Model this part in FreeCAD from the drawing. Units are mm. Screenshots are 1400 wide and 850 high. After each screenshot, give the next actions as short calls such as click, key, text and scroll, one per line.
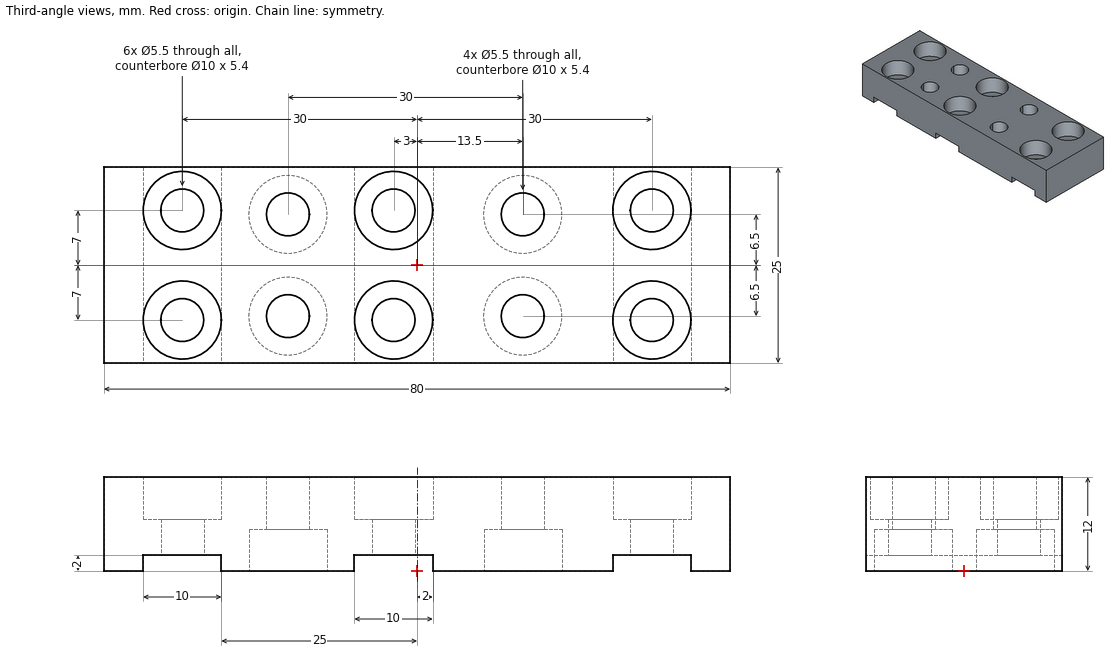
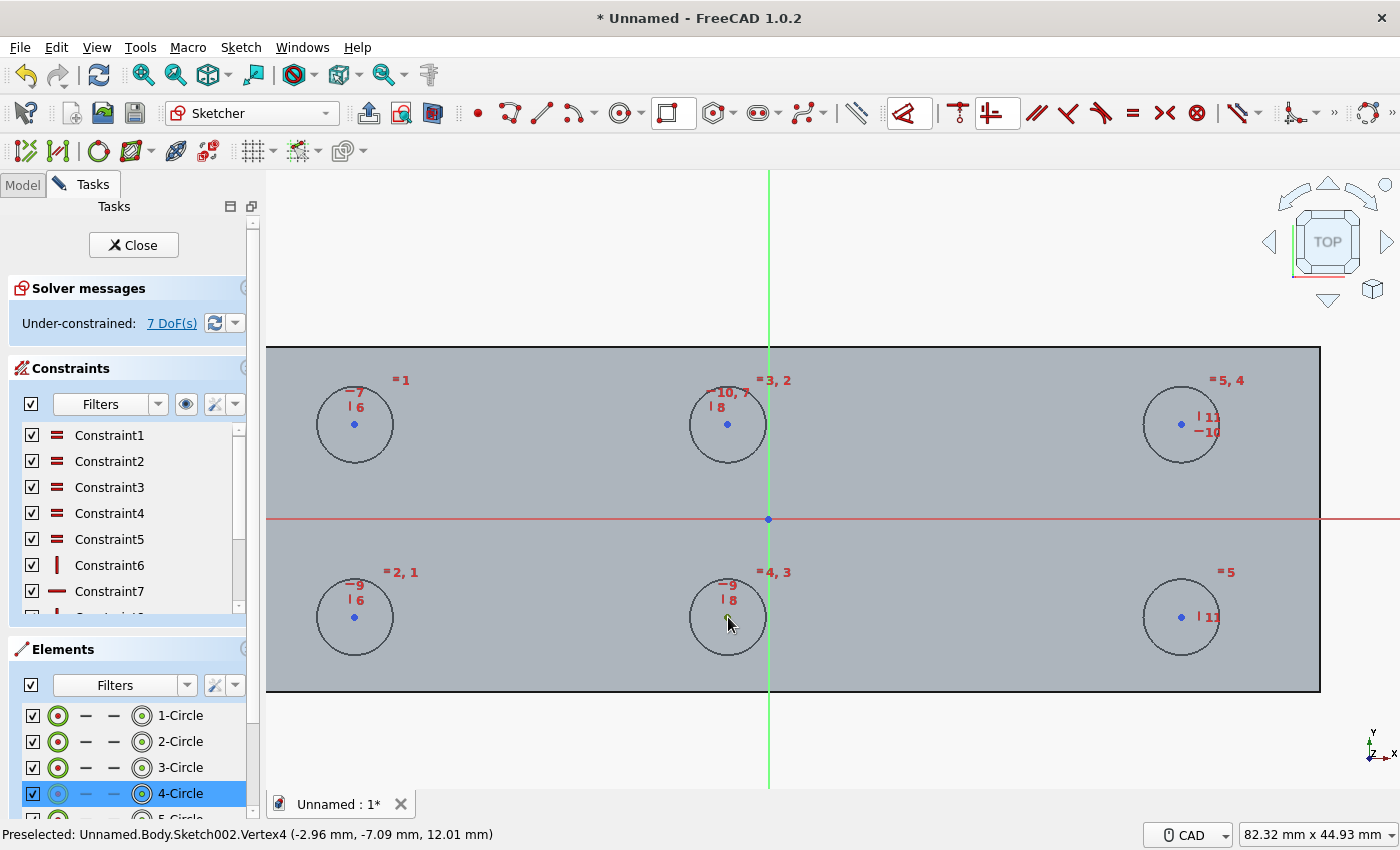
click(1181, 617)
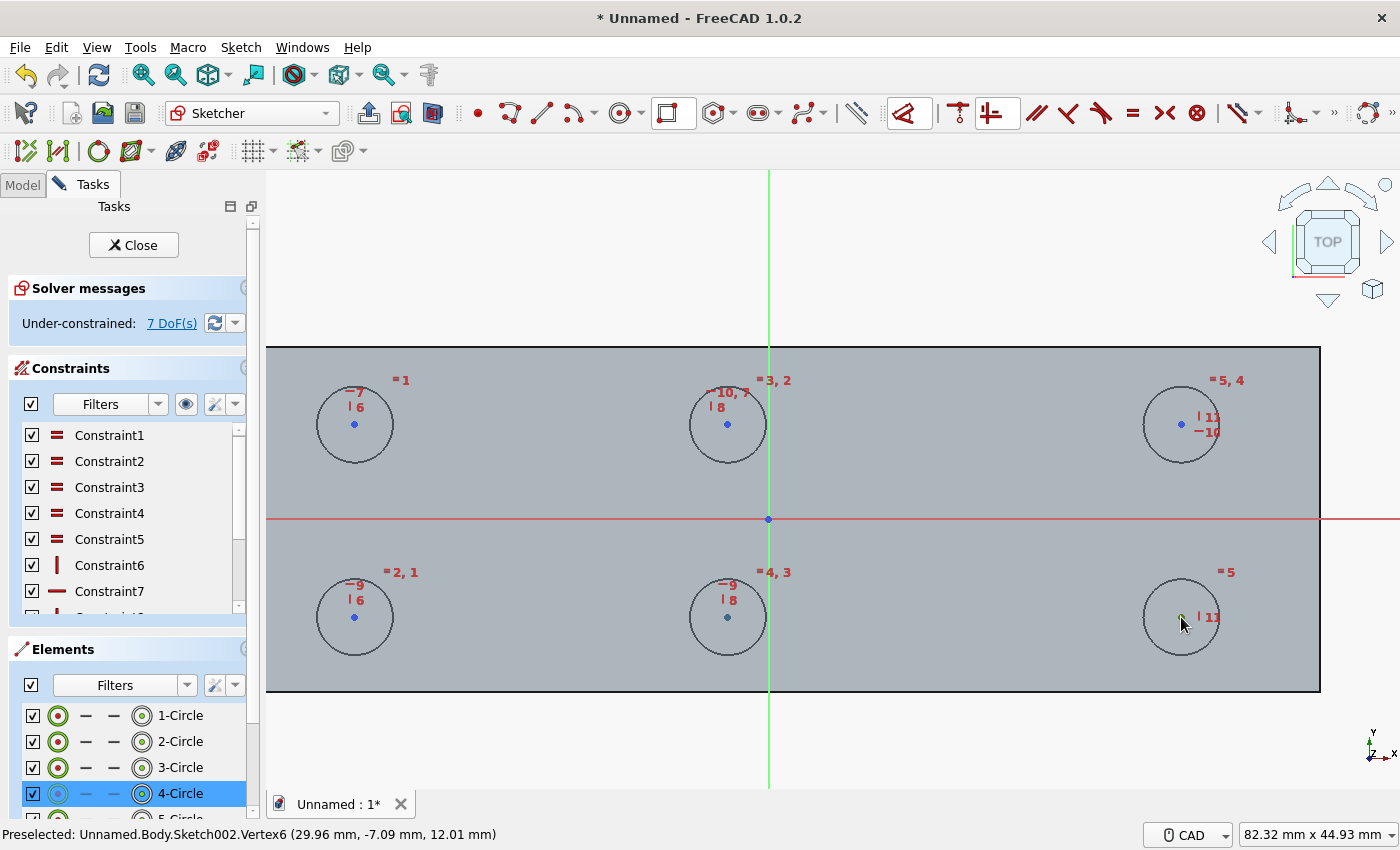
click(1014, 114)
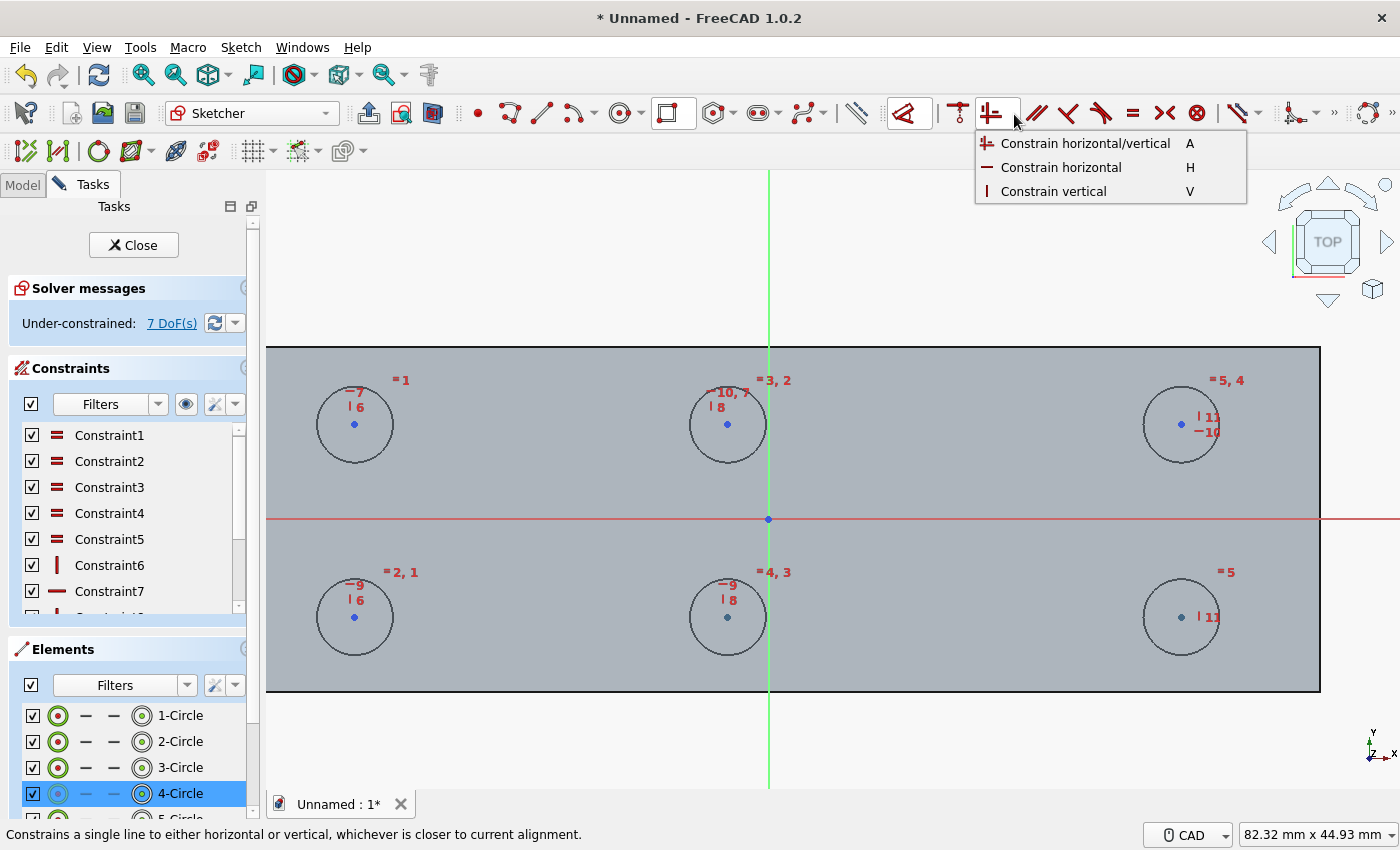
click(1111, 167)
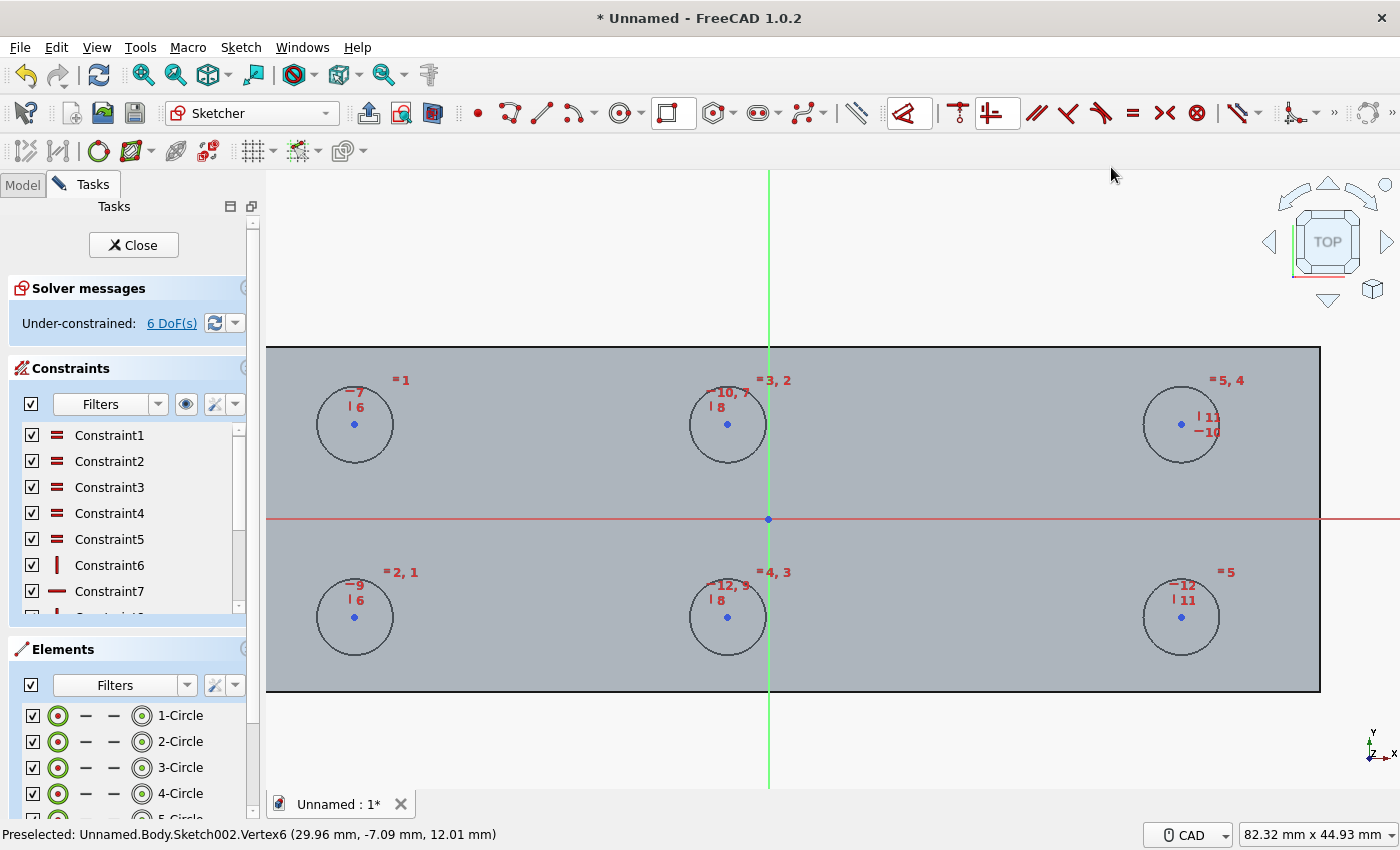
click(382, 398)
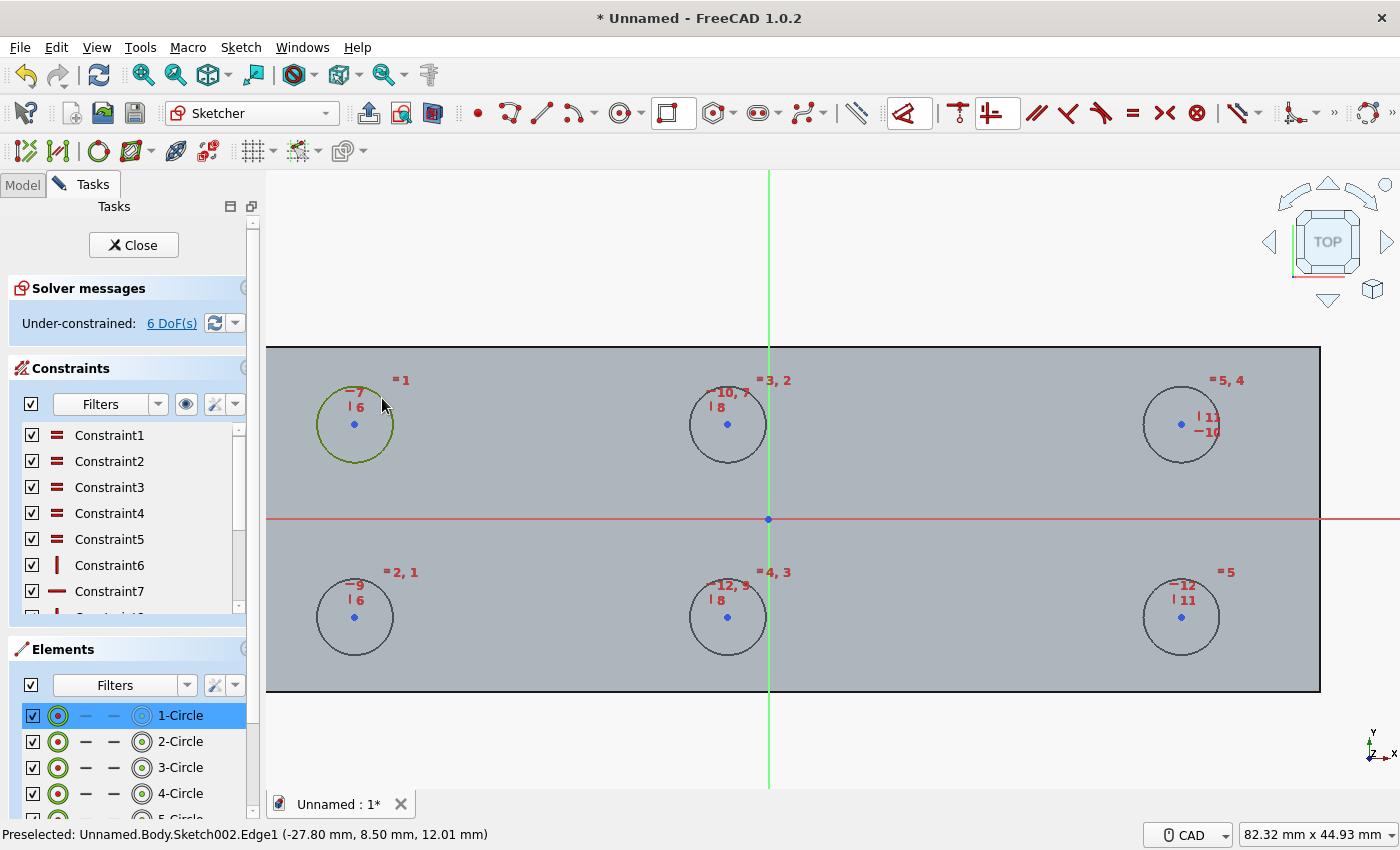
click(926, 114)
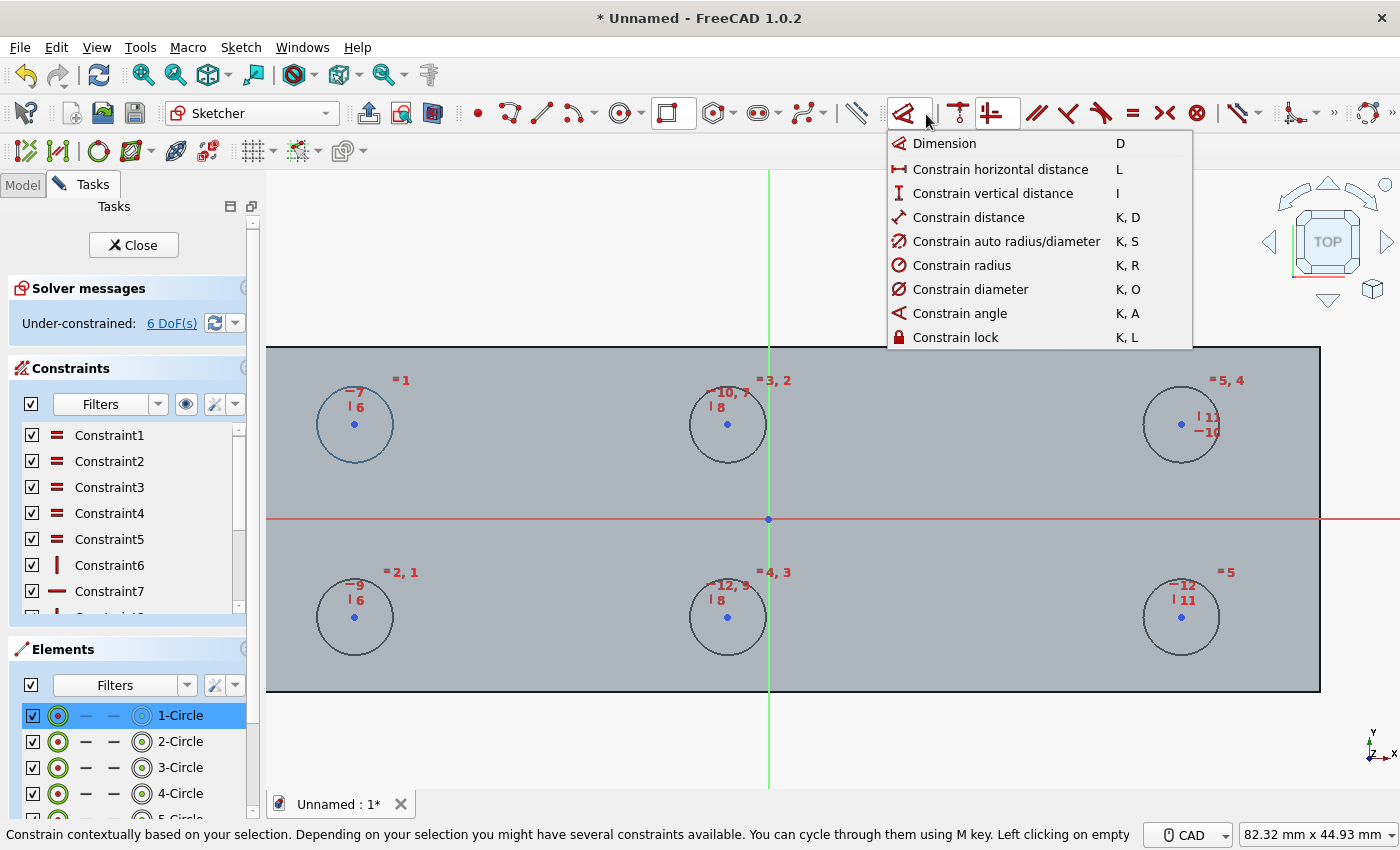
click(1040, 289)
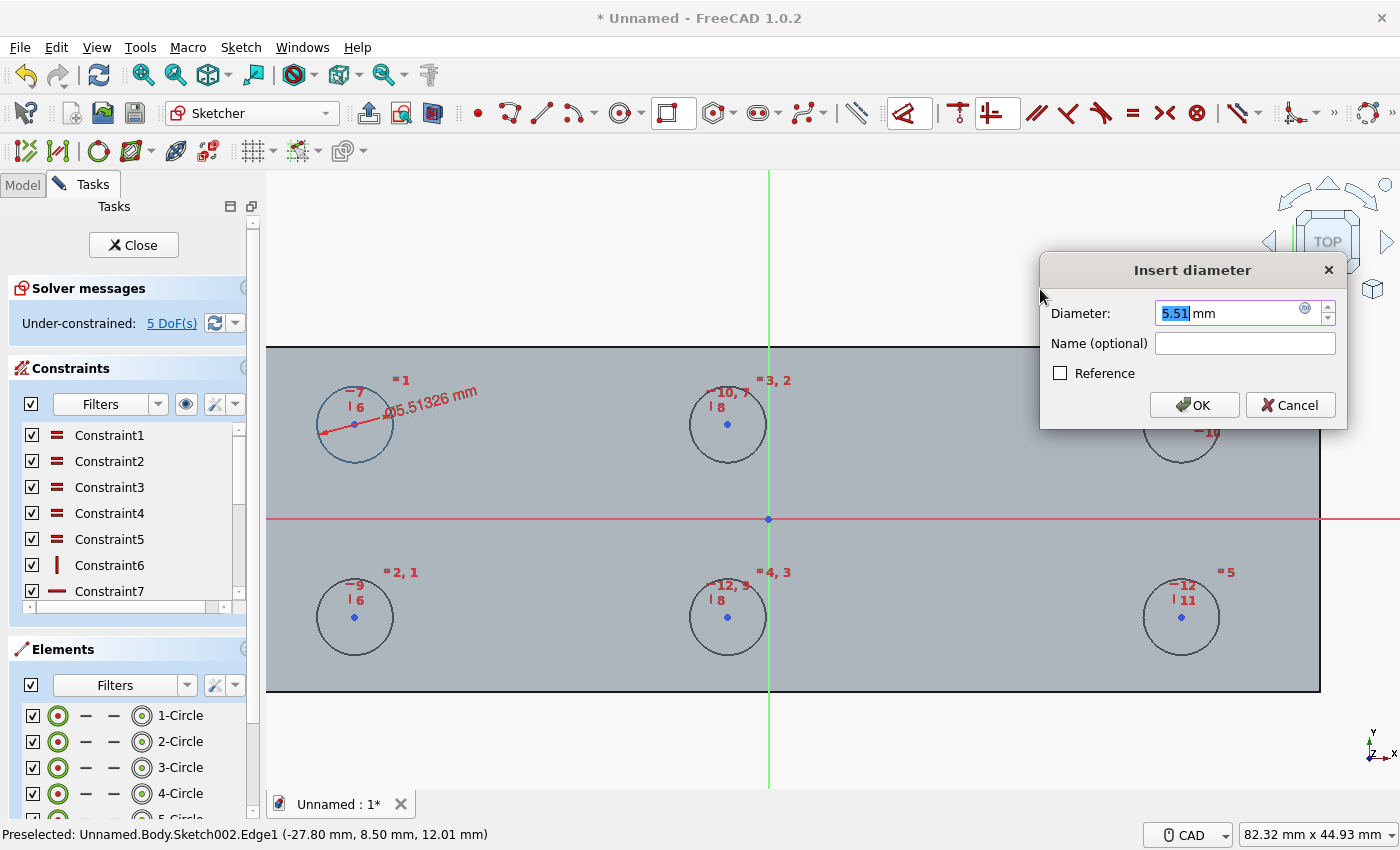
text(5.5)
key(Return)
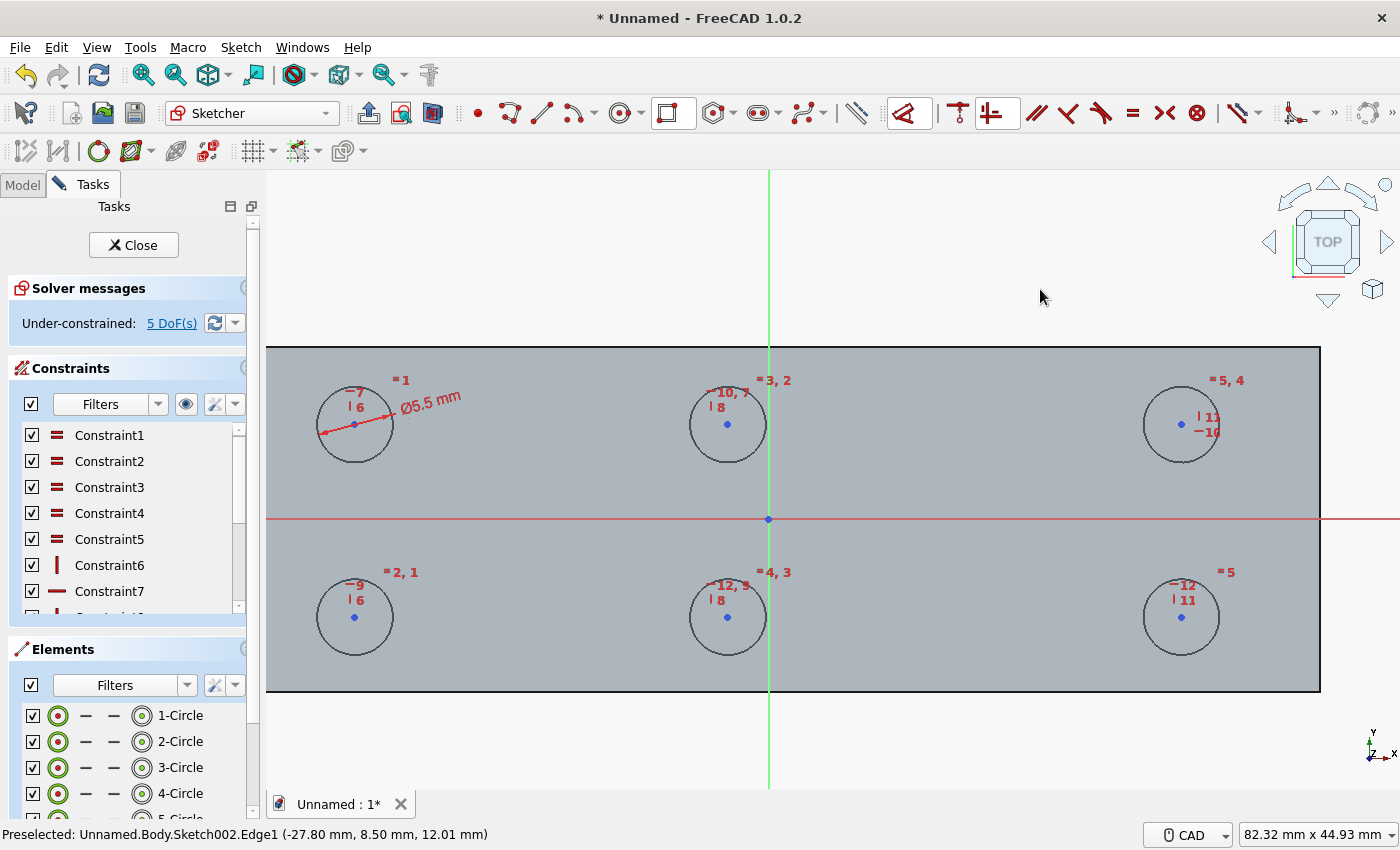
click(355, 425)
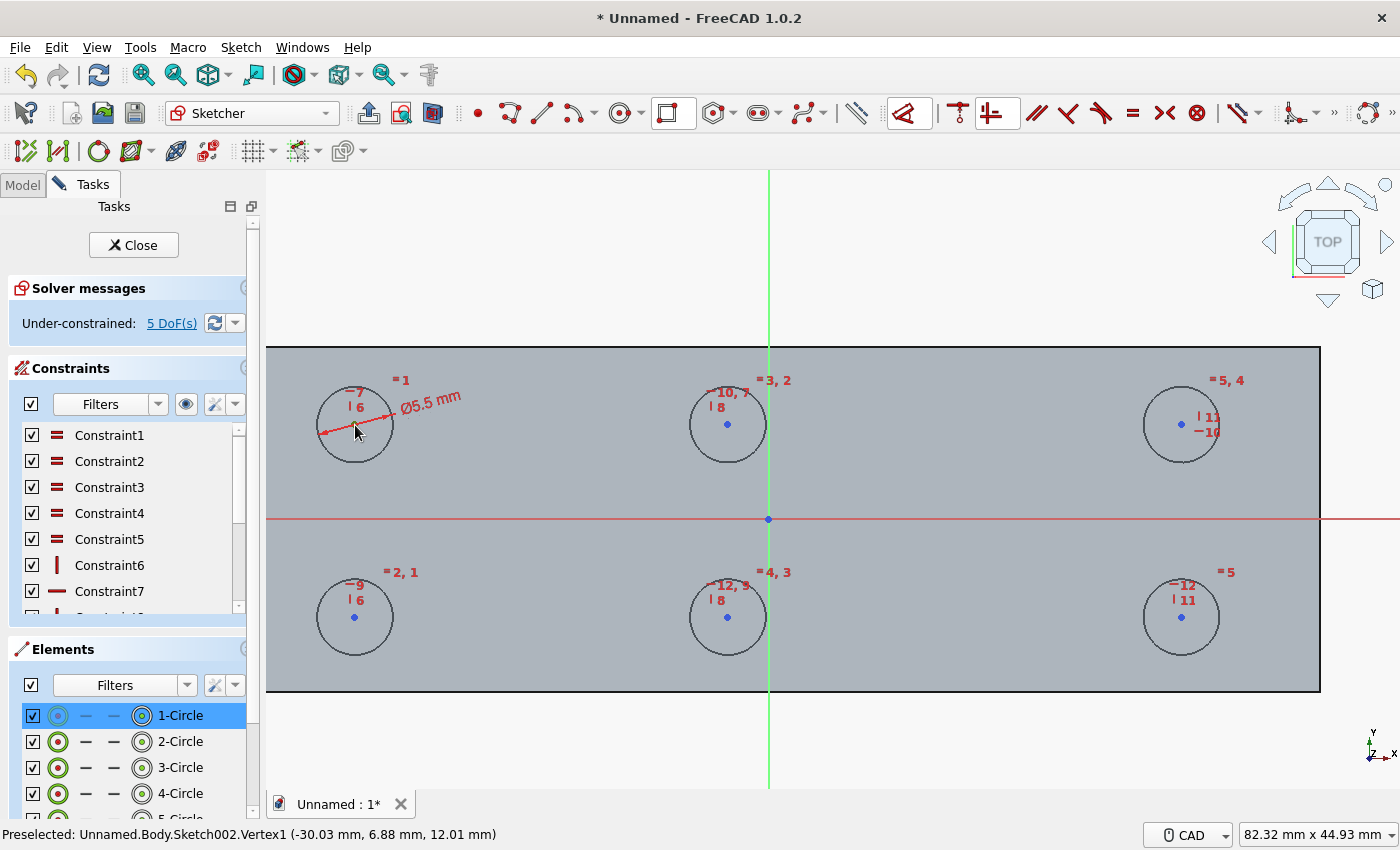
click(926, 114)